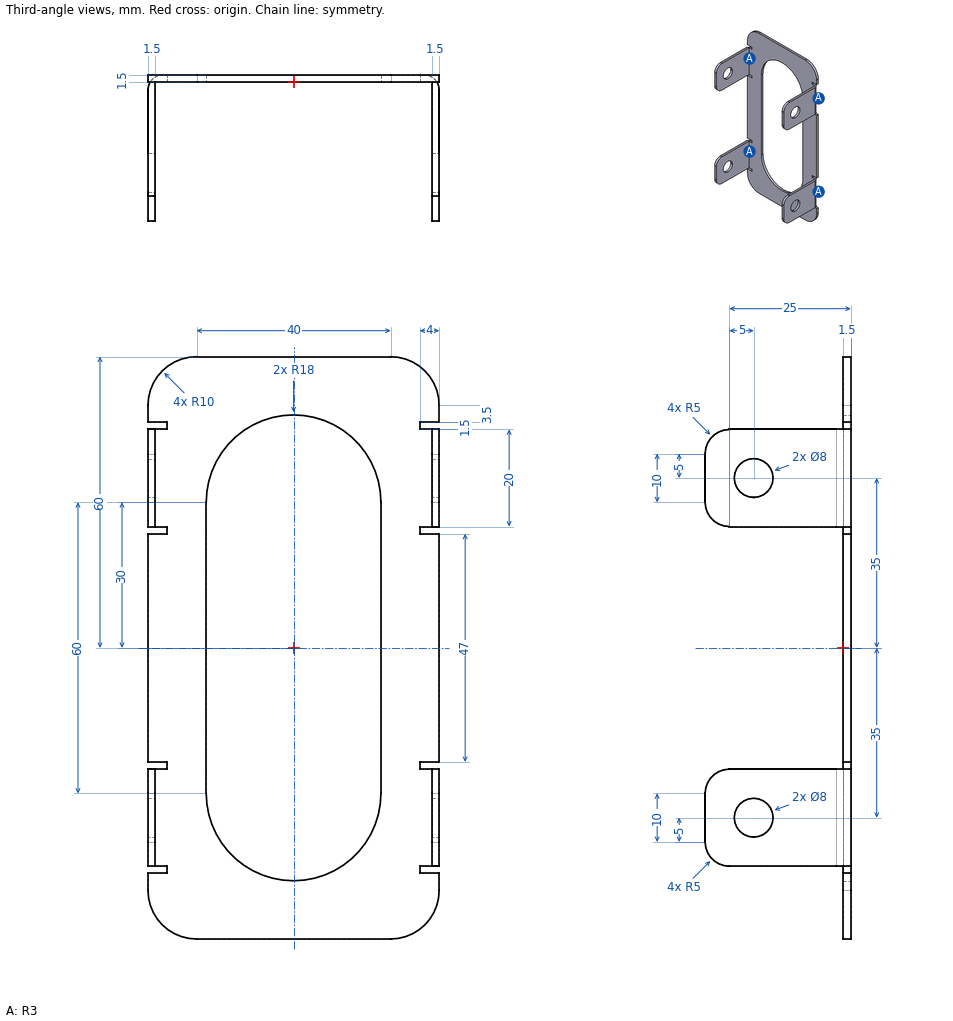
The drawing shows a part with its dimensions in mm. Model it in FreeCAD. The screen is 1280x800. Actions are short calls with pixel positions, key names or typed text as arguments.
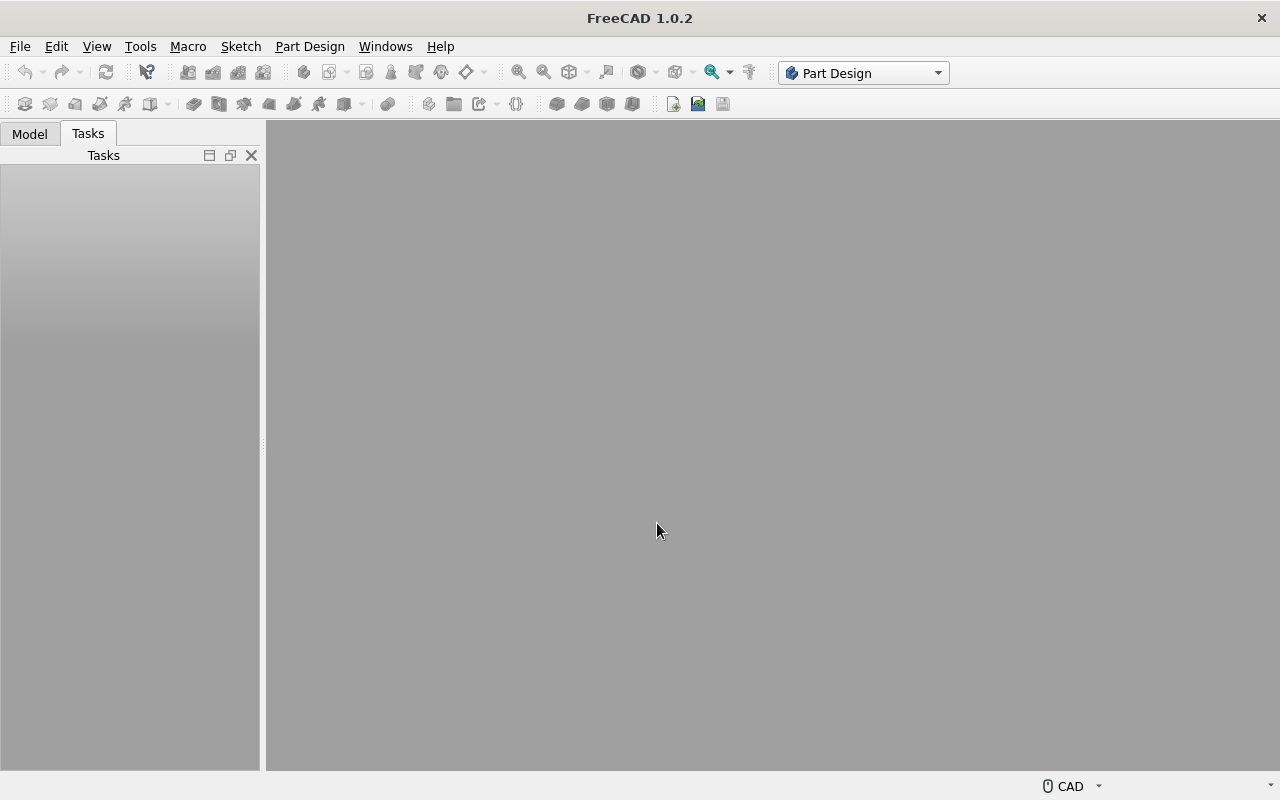
click(673, 104)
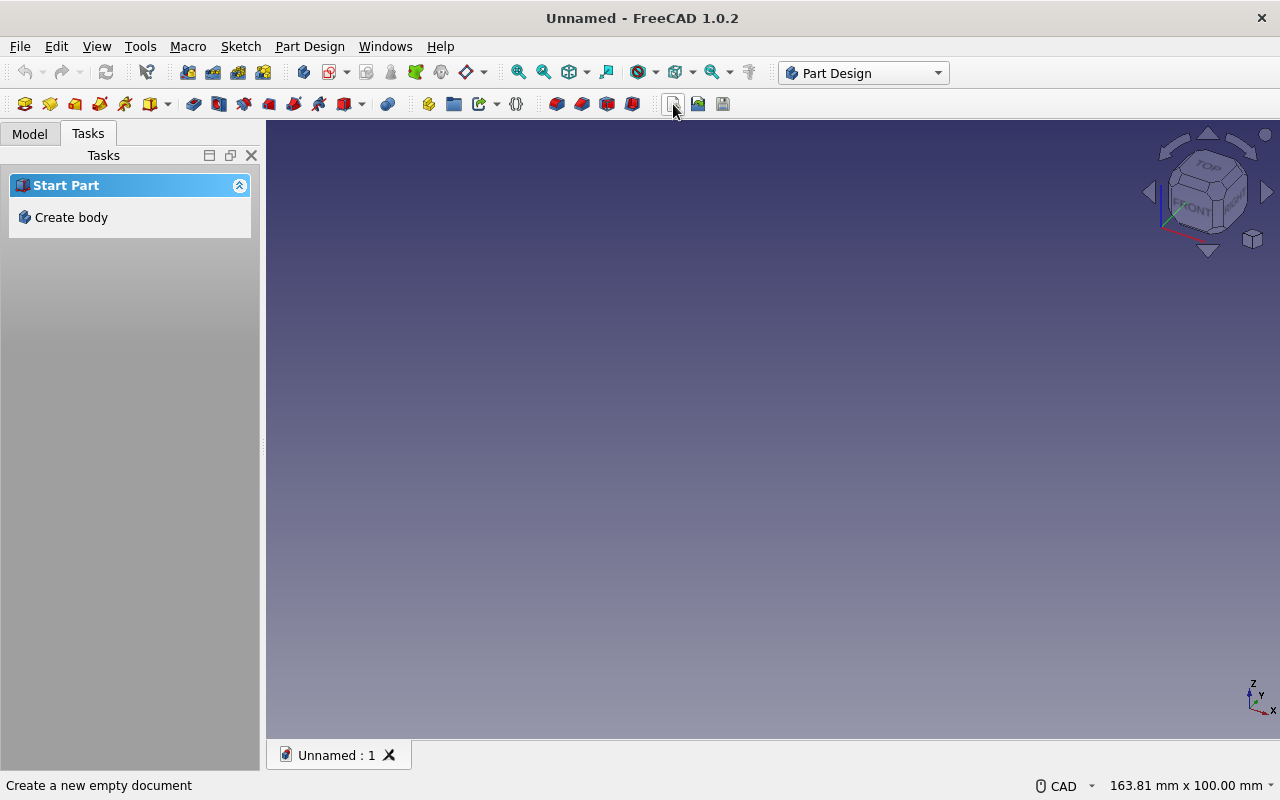
click(328, 72)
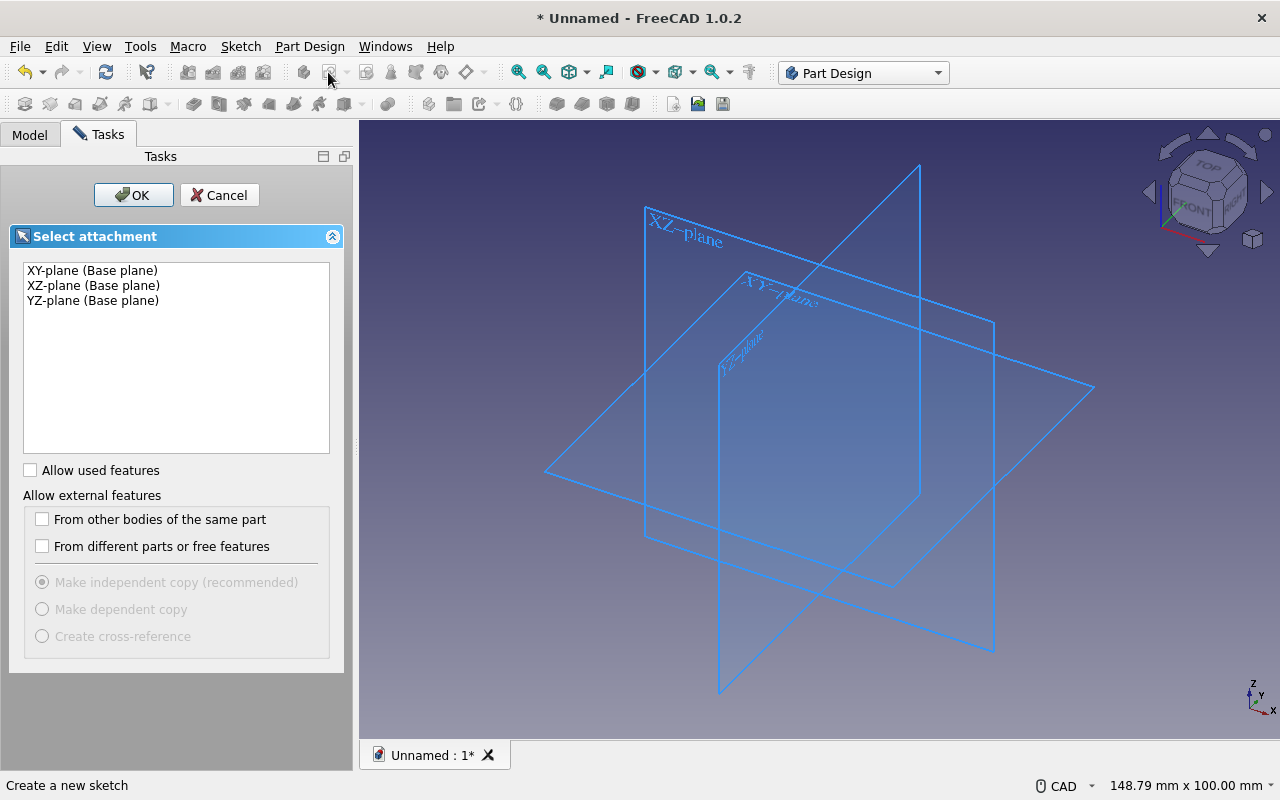
click(84, 286)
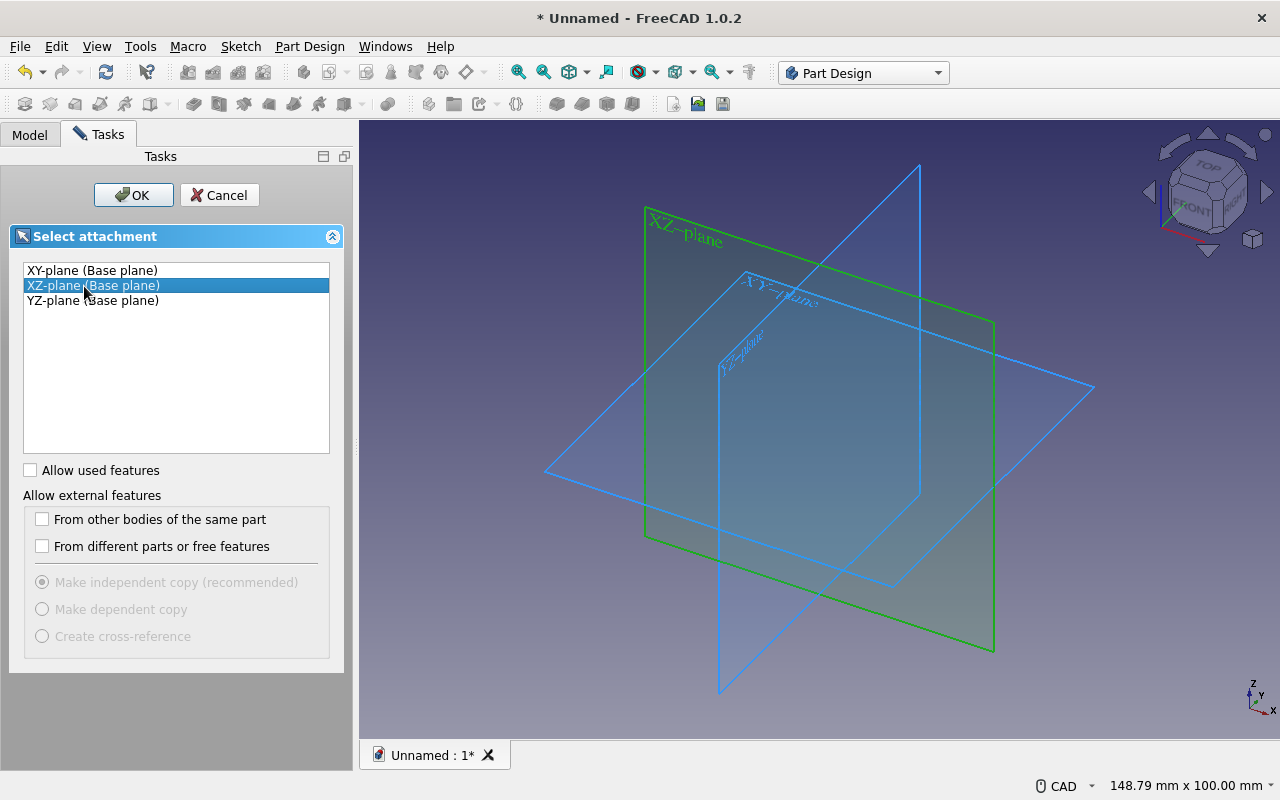
click(134, 195)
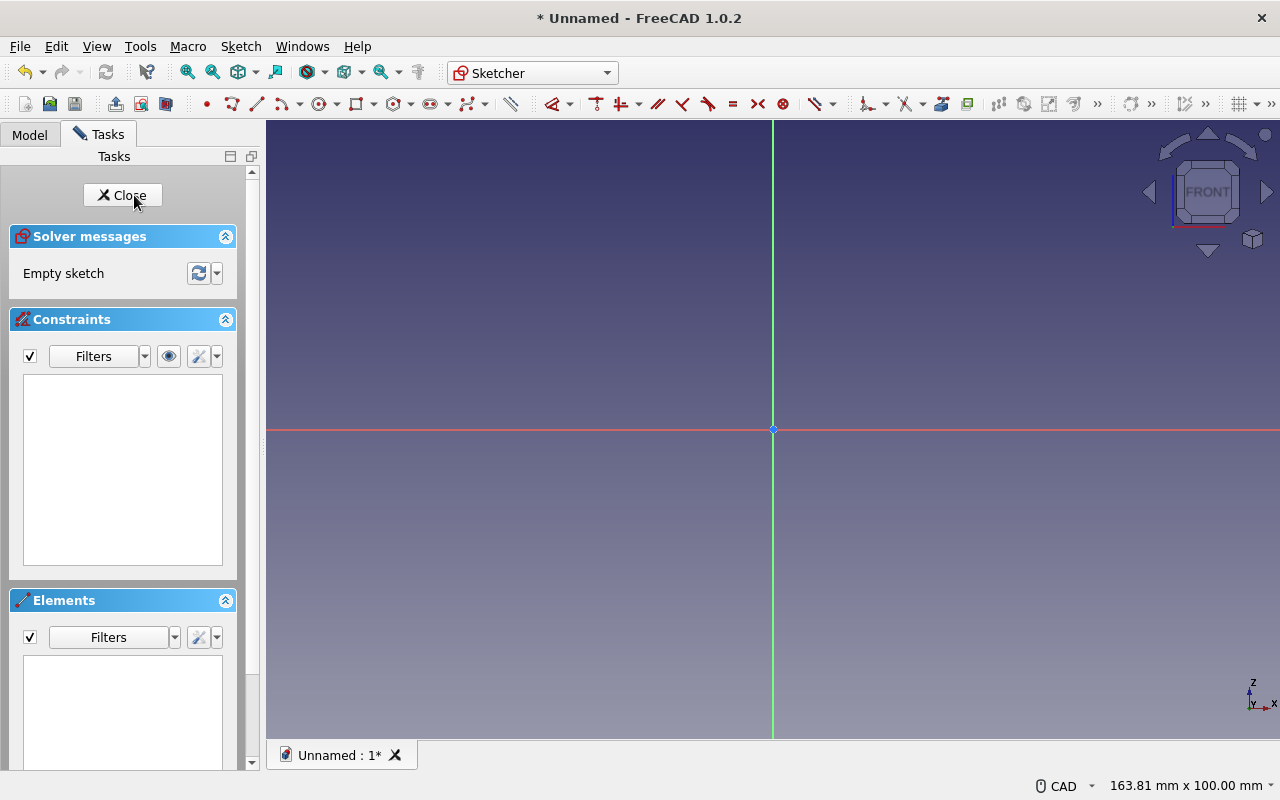
scroll(621, 430, down, 3)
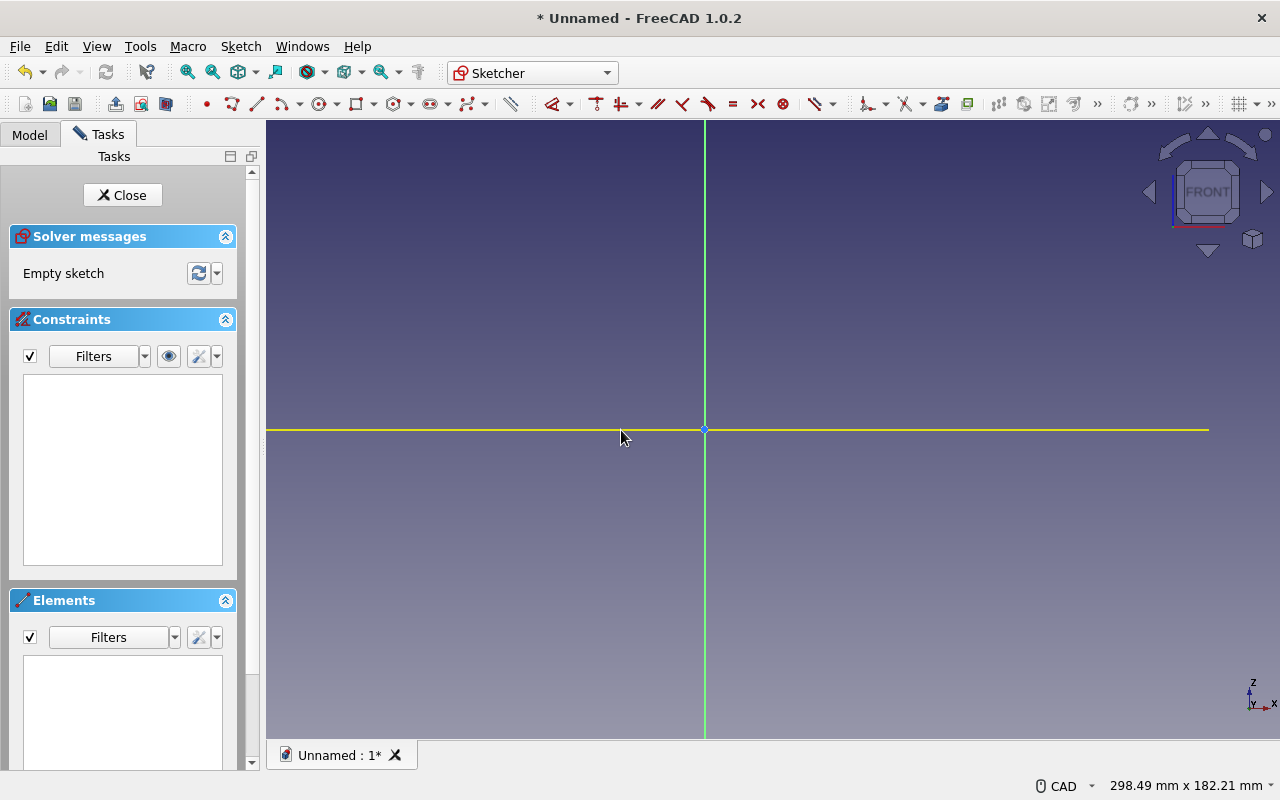
click(257, 104)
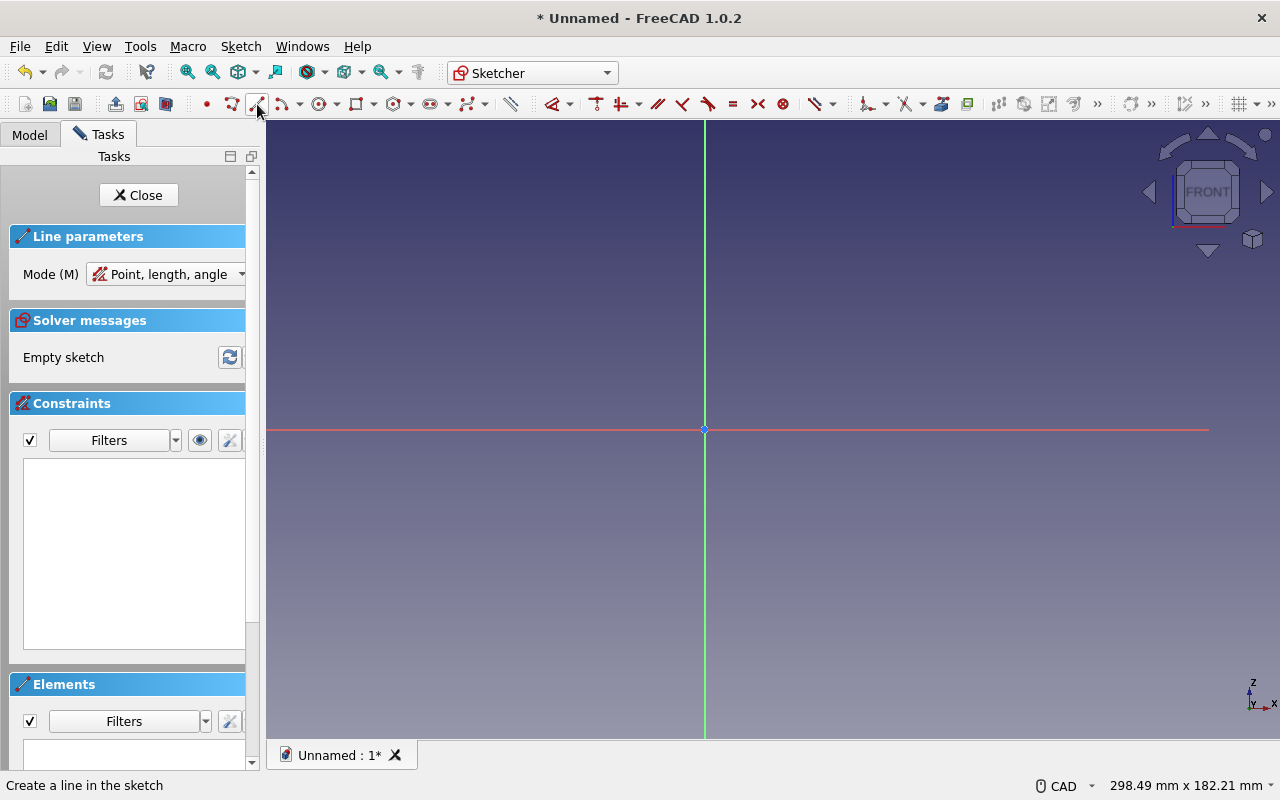
click(637, 226)
click(773, 226)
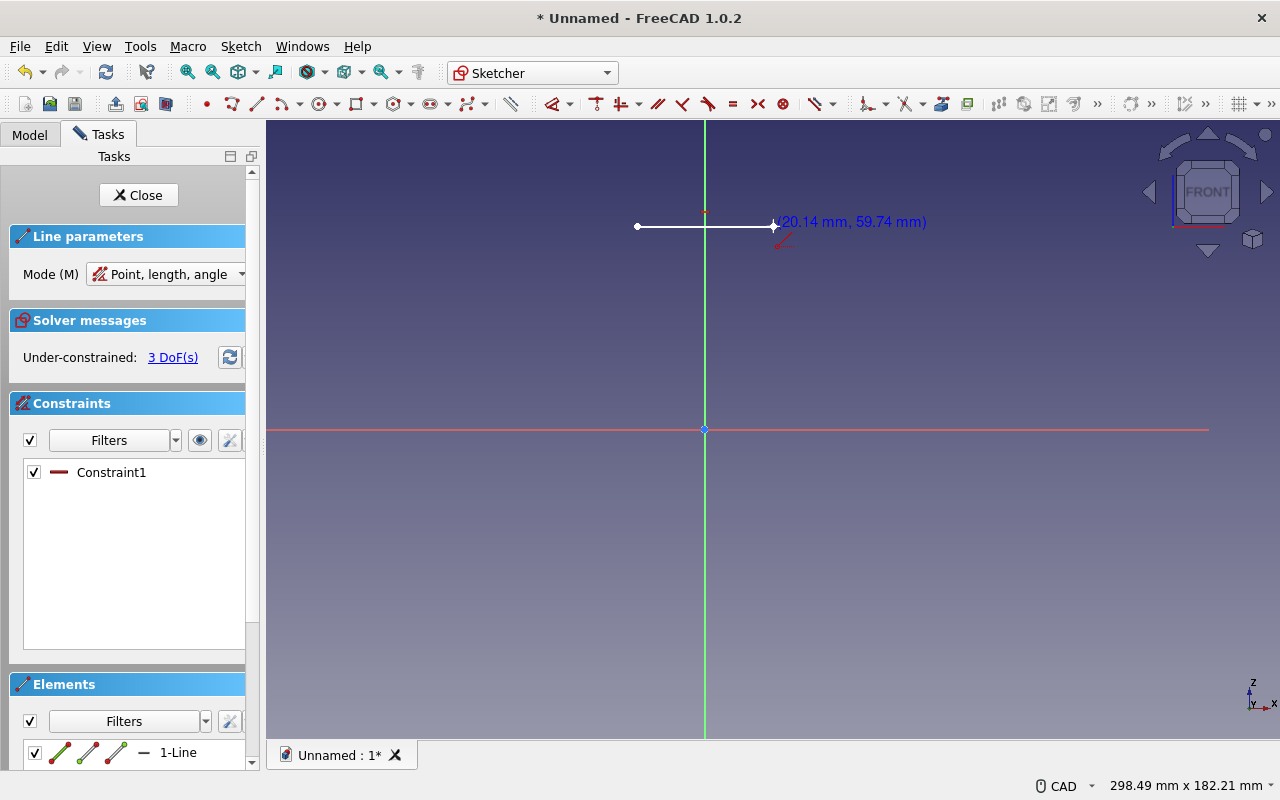
click(232, 104)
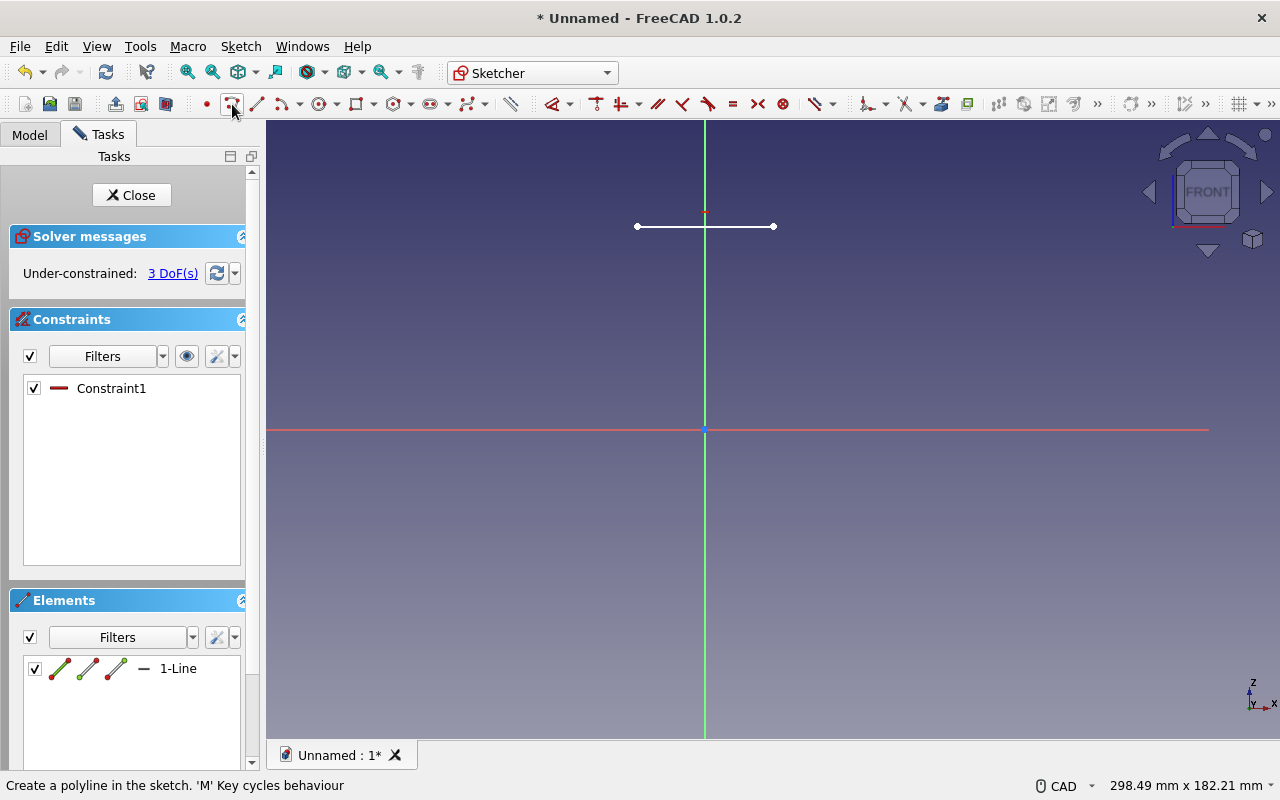
click(806, 260)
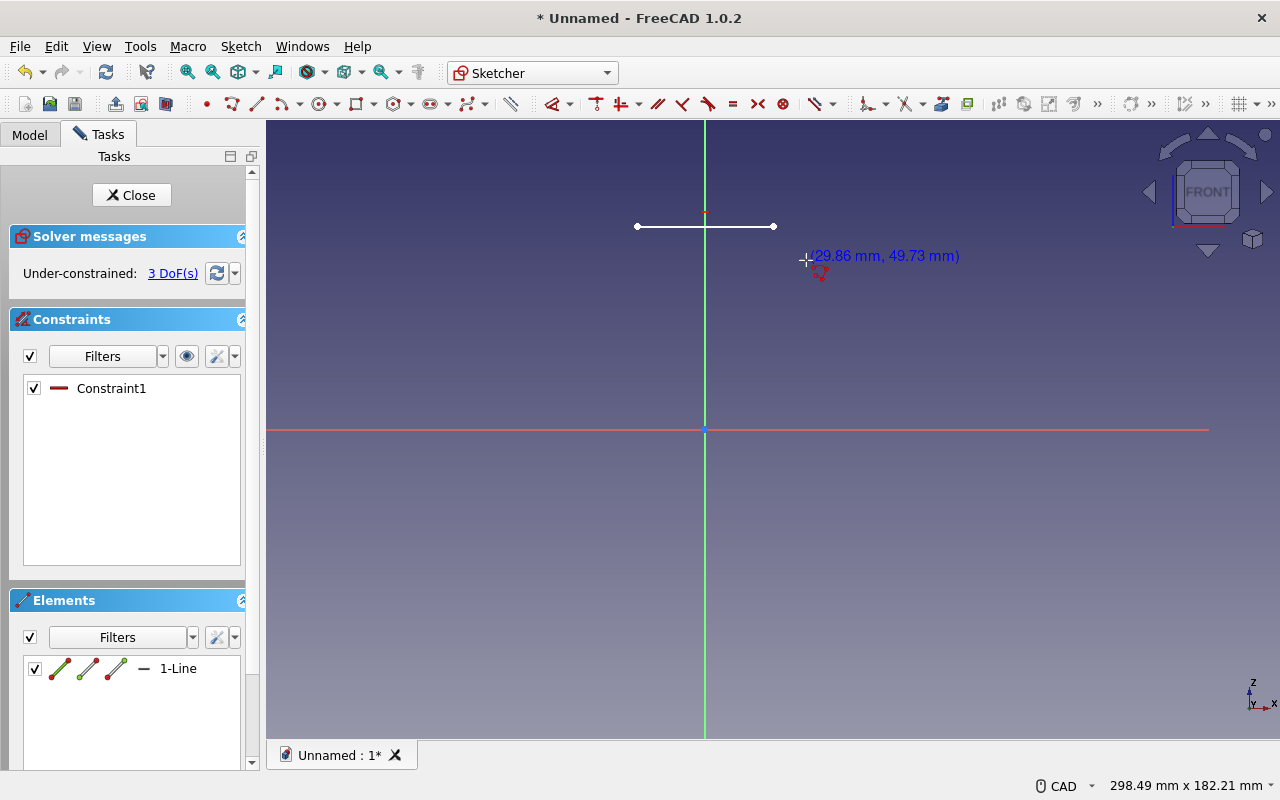
scroll(806, 272, up, 2)